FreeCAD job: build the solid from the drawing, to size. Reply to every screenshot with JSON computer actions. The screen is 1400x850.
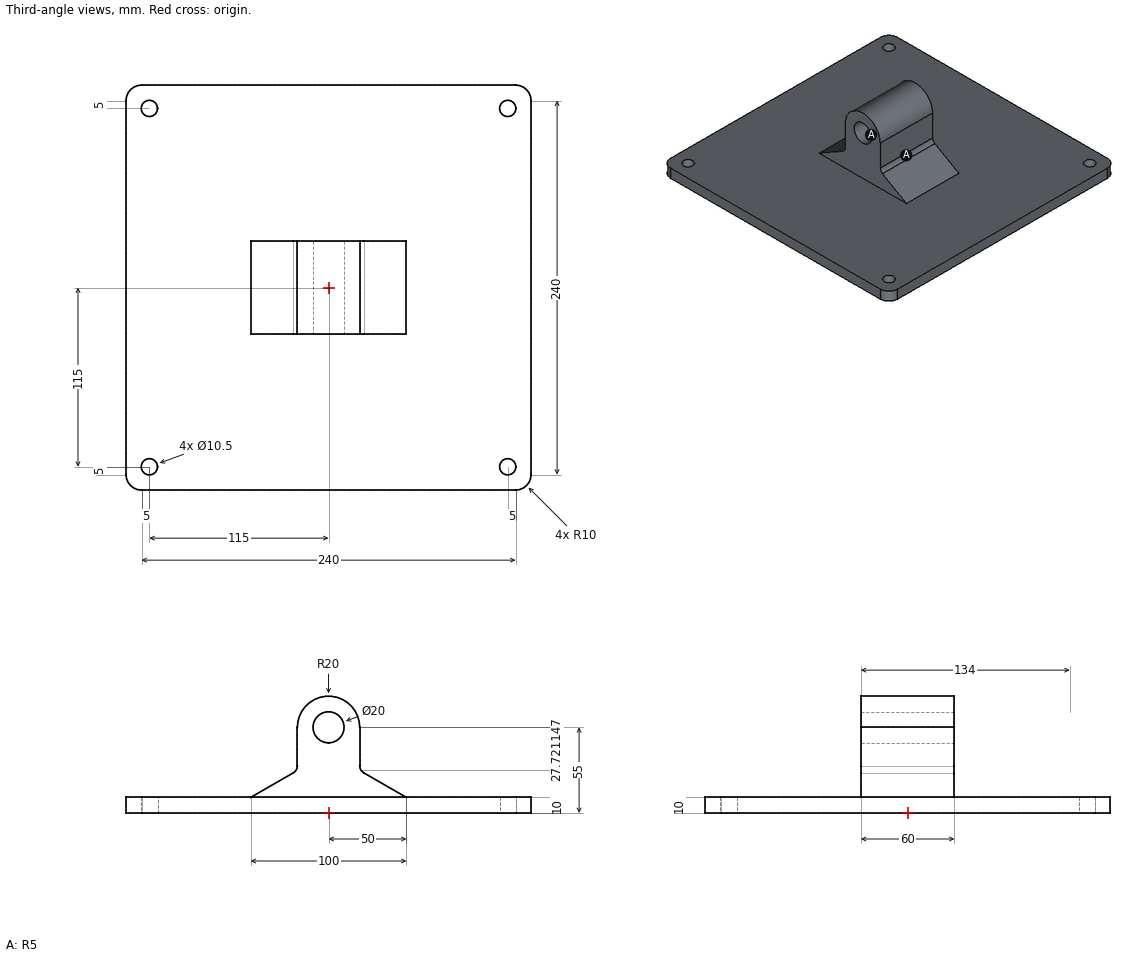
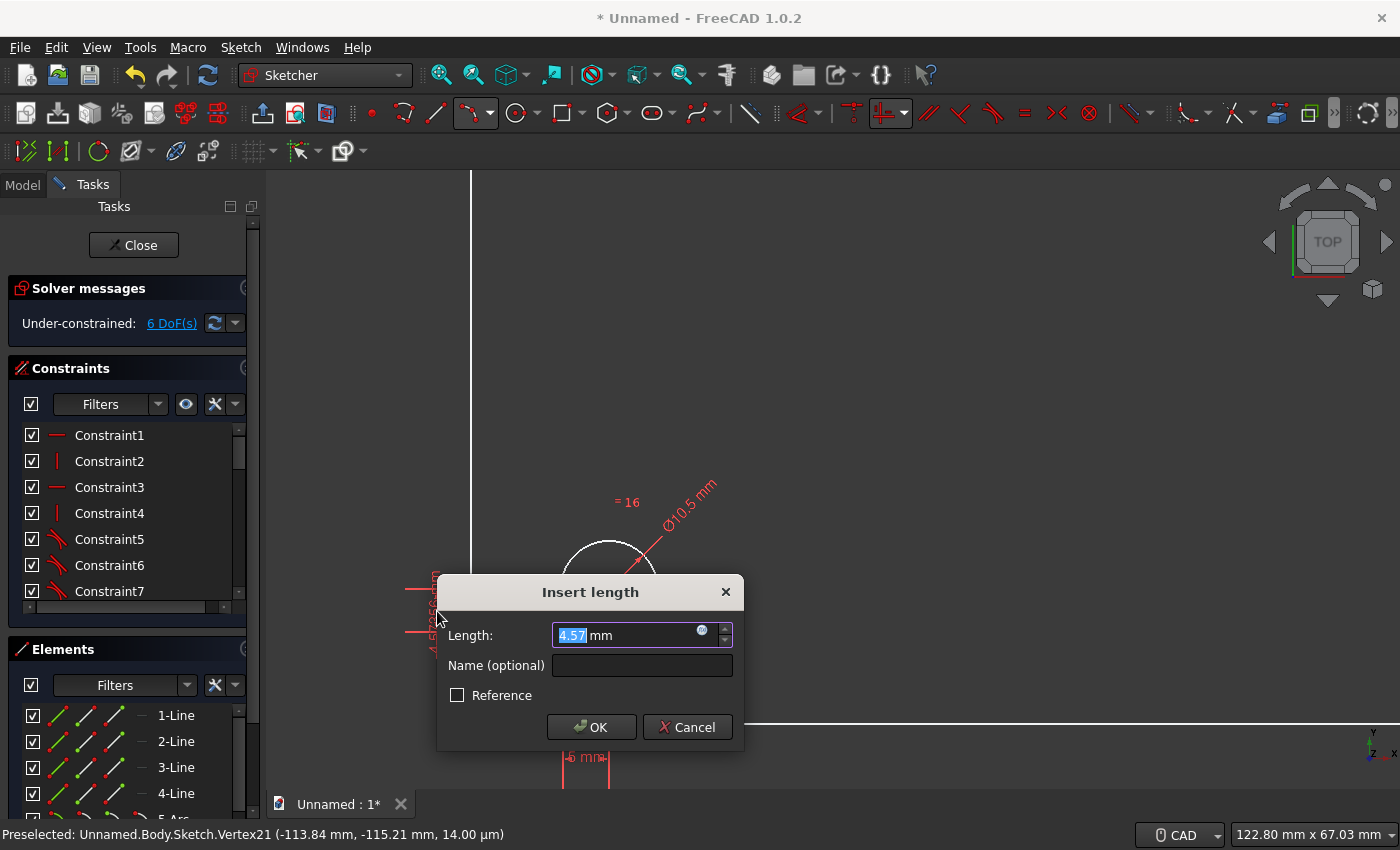
{"action": "type", "text": "5"}
{"action": "key", "text": "Return"}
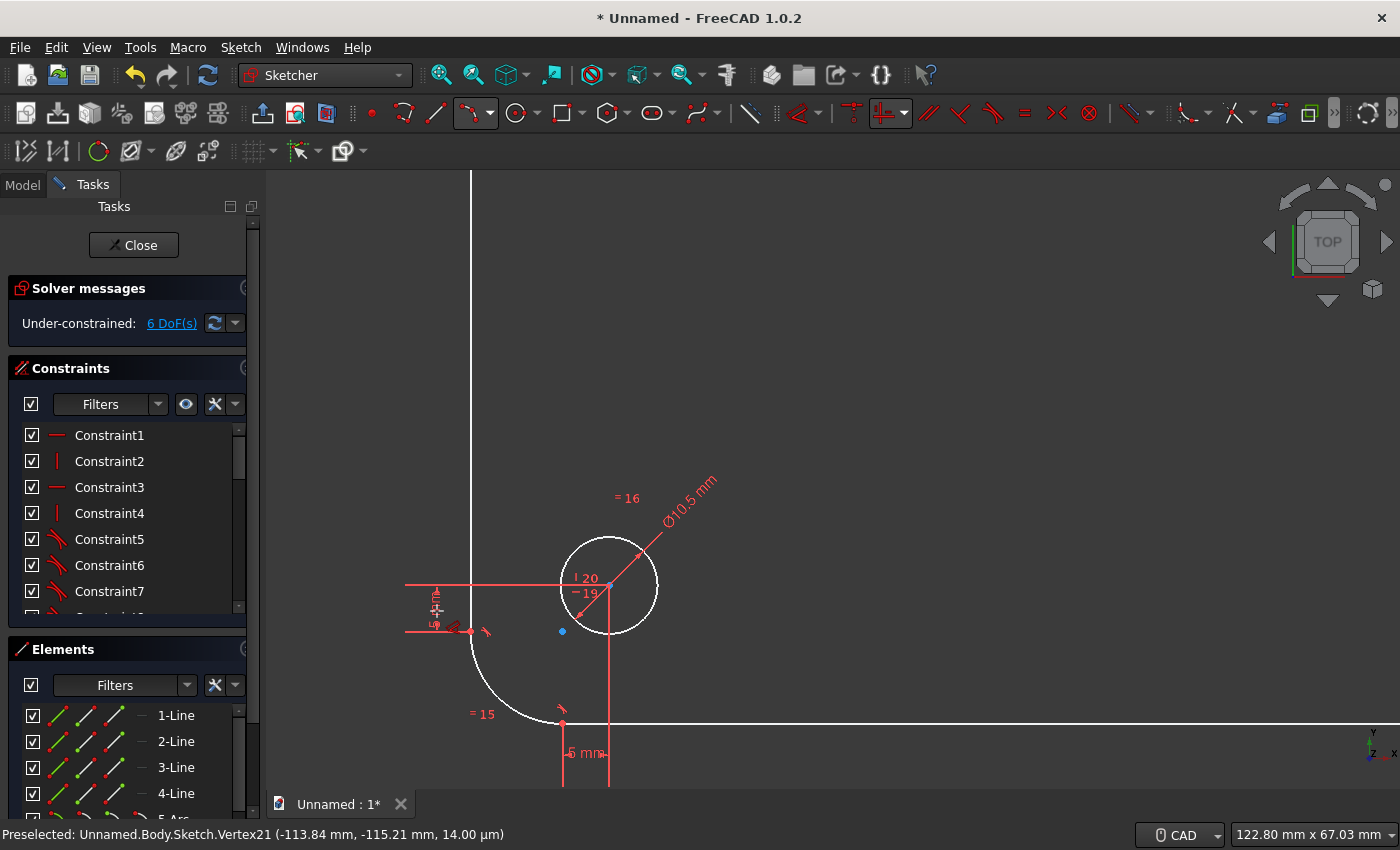
{"action": "scroll", "coordinate": [587, 668], "scroll_direction": "down", "scroll_amount": 9}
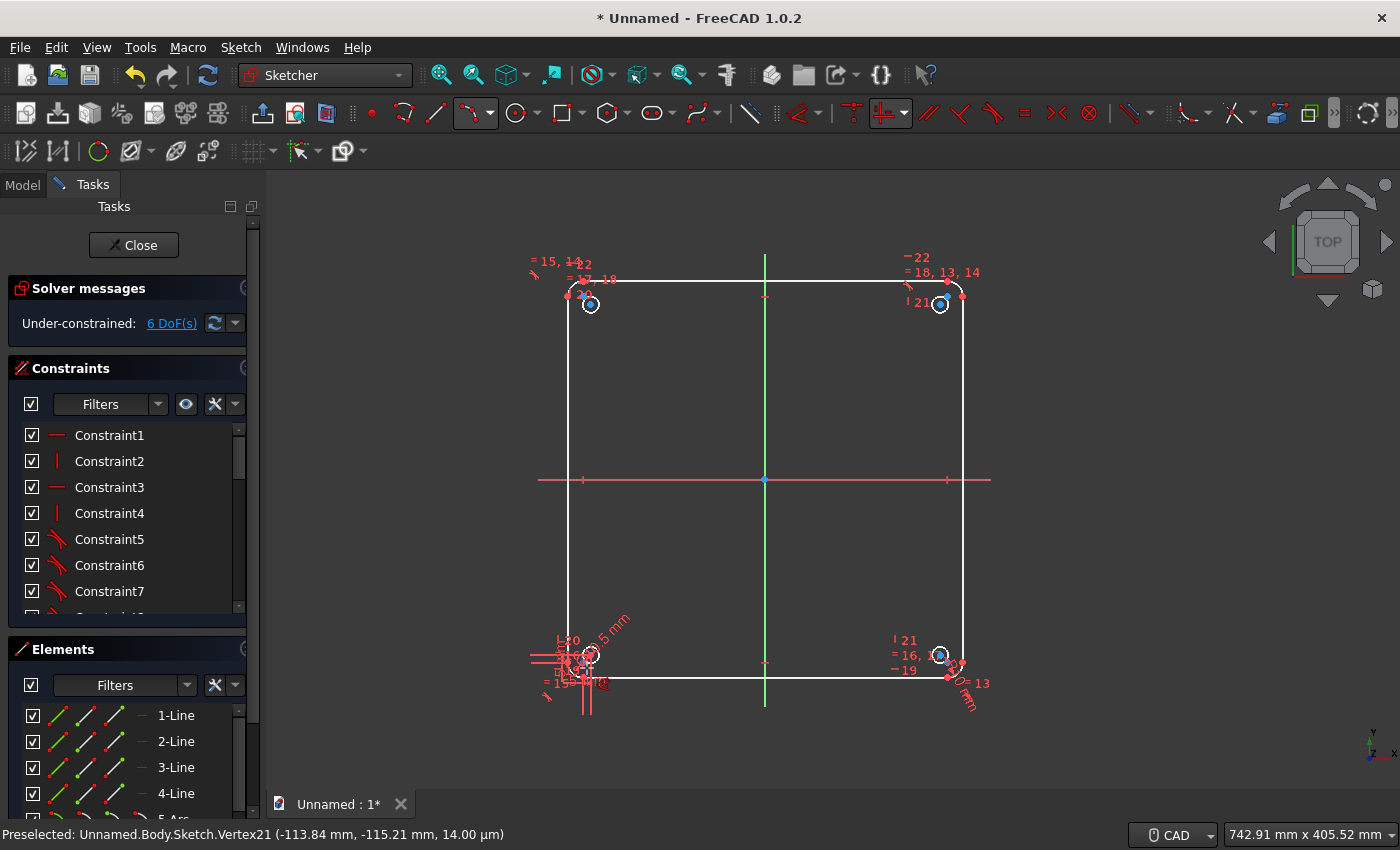
{"action": "scroll", "coordinate": [948, 678], "scroll_direction": "up", "scroll_amount": 9}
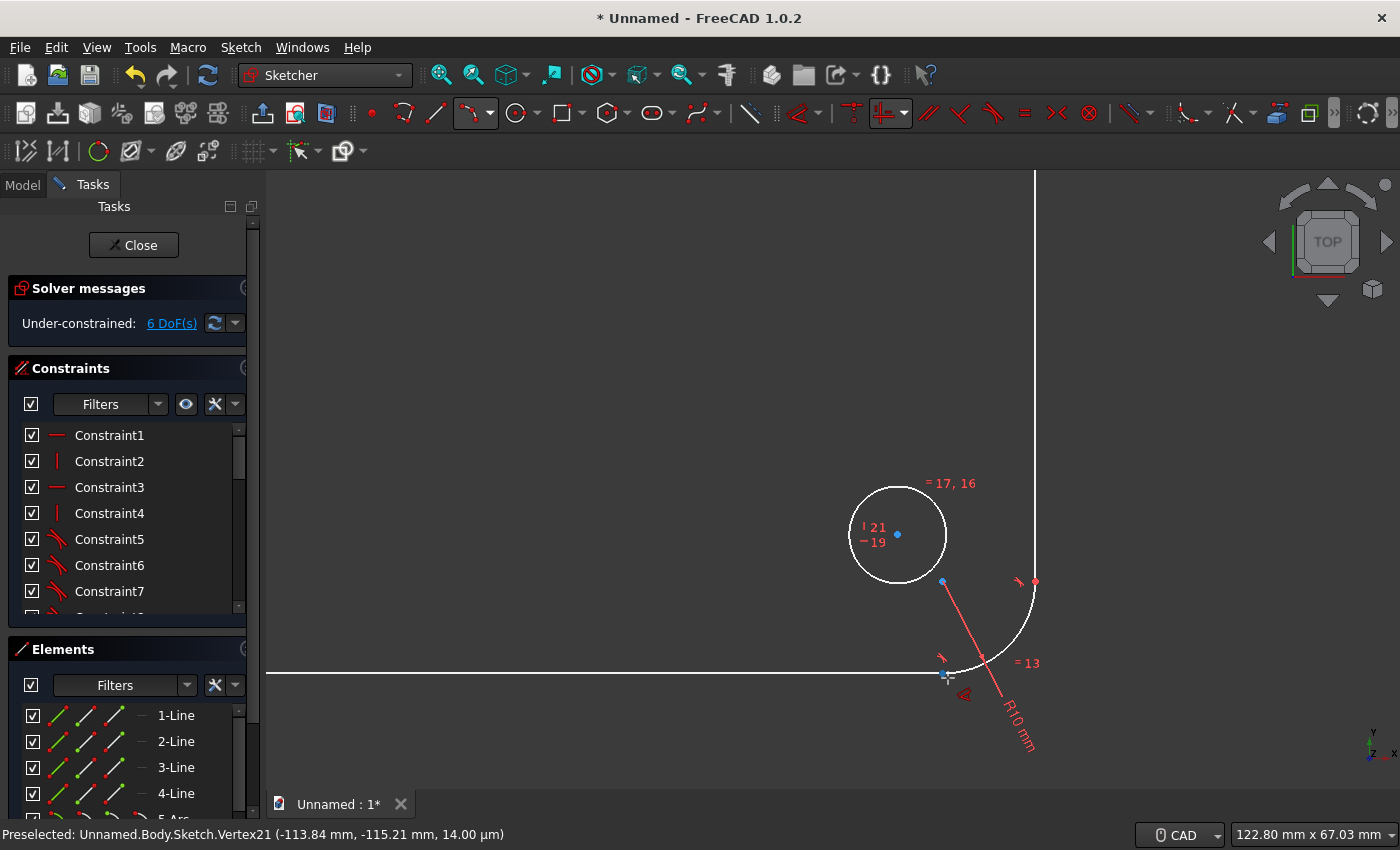
{"action": "left_click", "coordinate": [943, 673]}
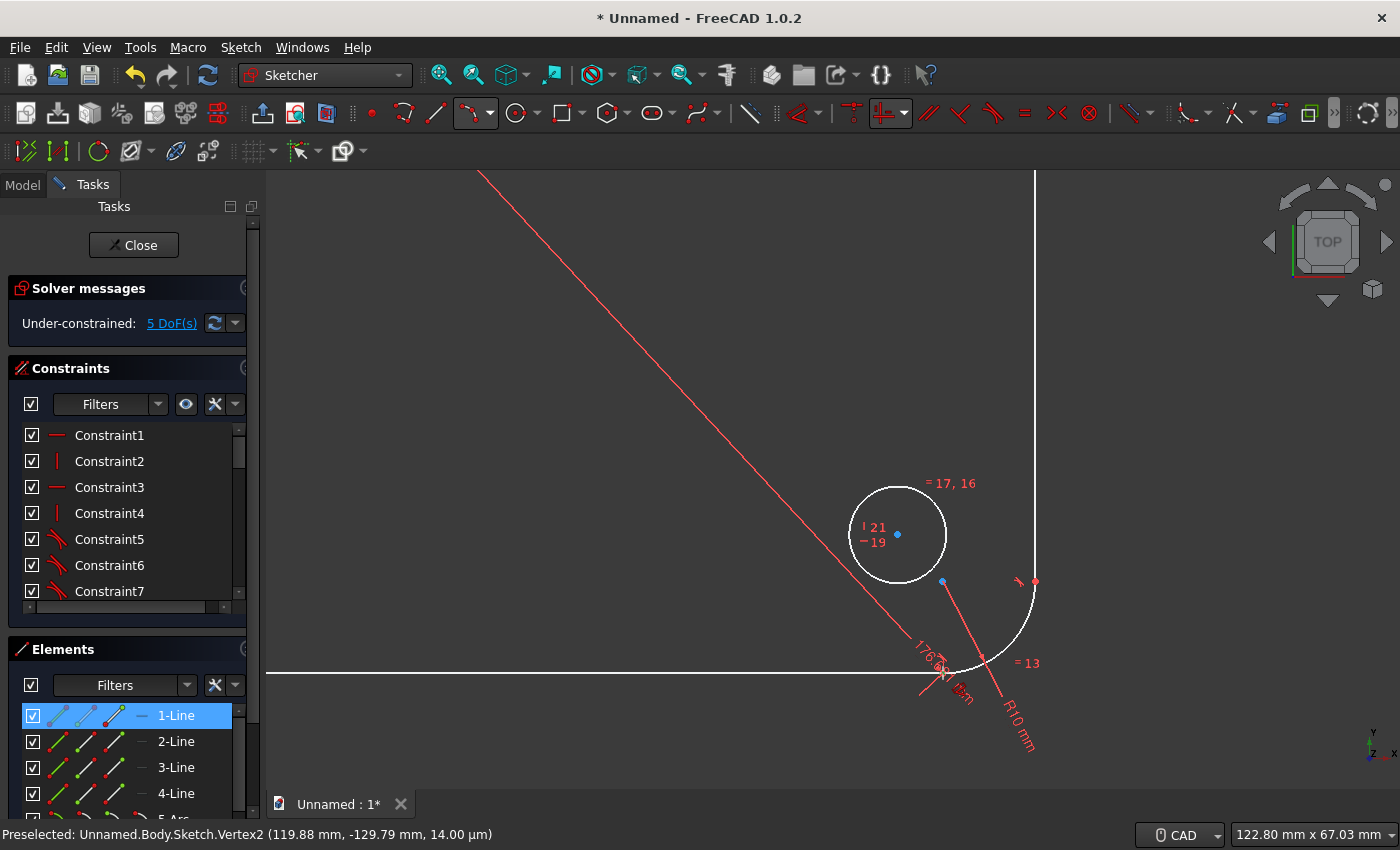
{"action": "left_click", "coordinate": [898, 535]}
{"action": "left_click", "coordinate": [920, 707]}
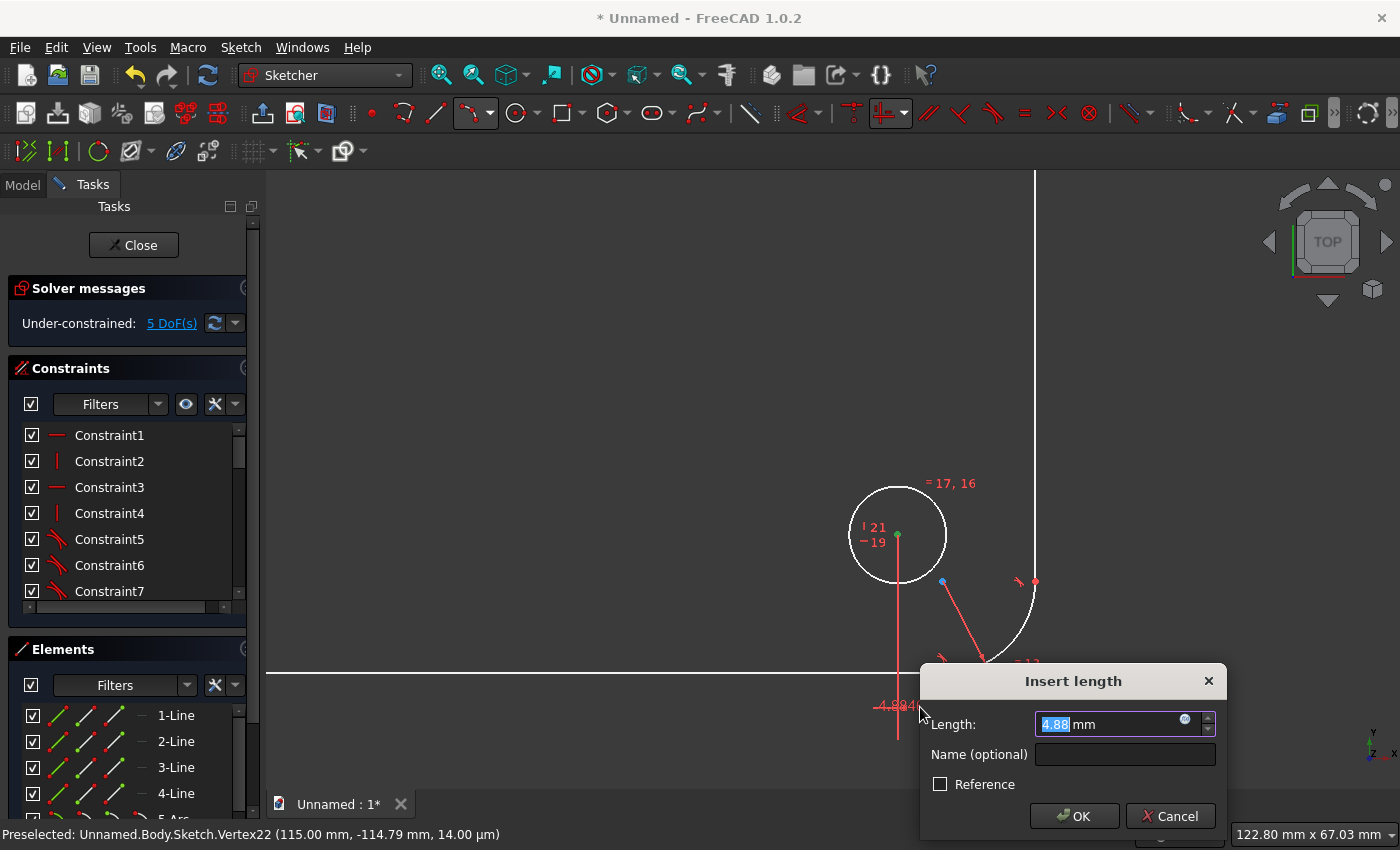
{"action": "type", "text": "5"}
{"action": "key", "text": "Return"}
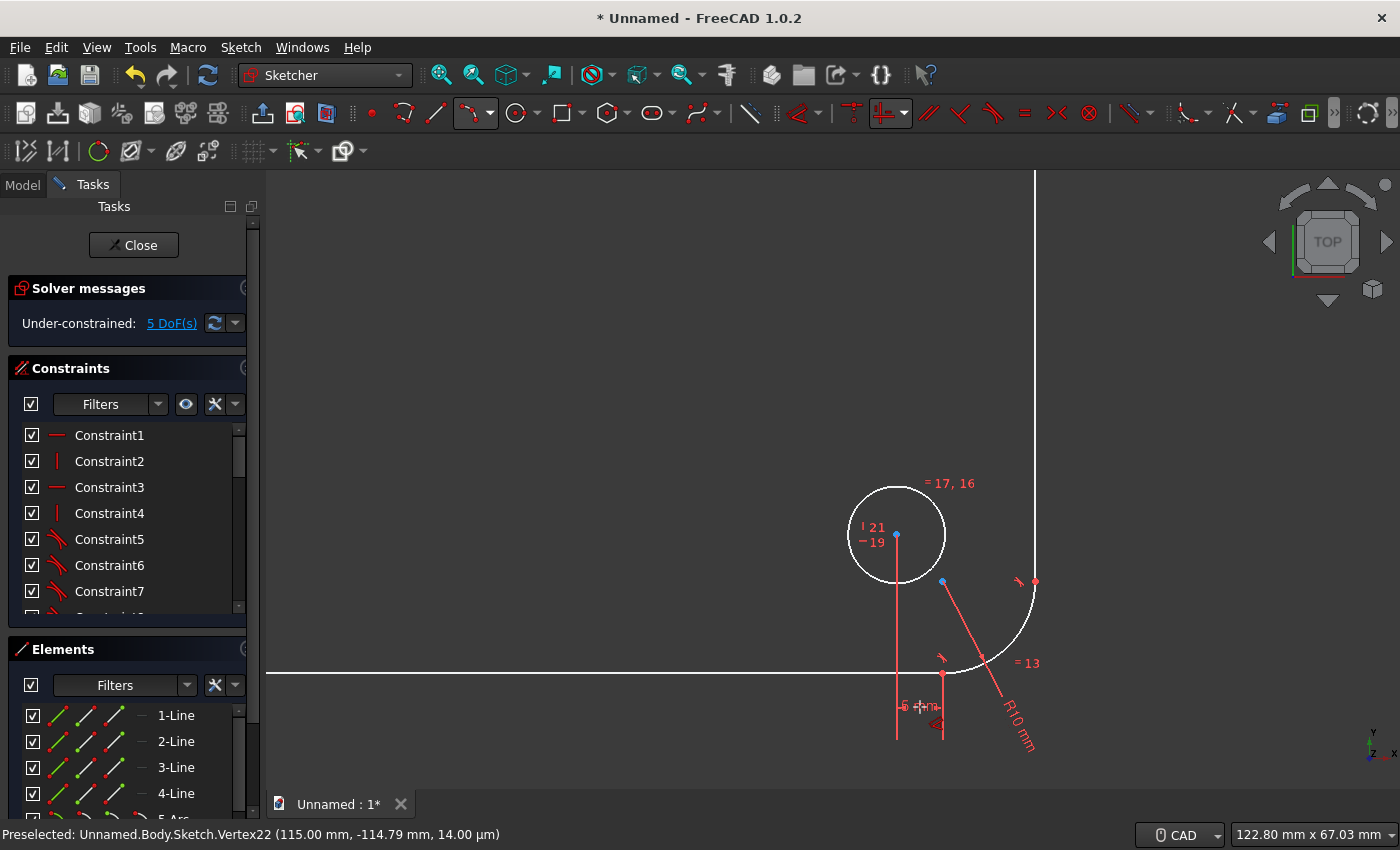
{"action": "scroll", "coordinate": [948, 678], "scroll_direction": "down", "scroll_amount": 9}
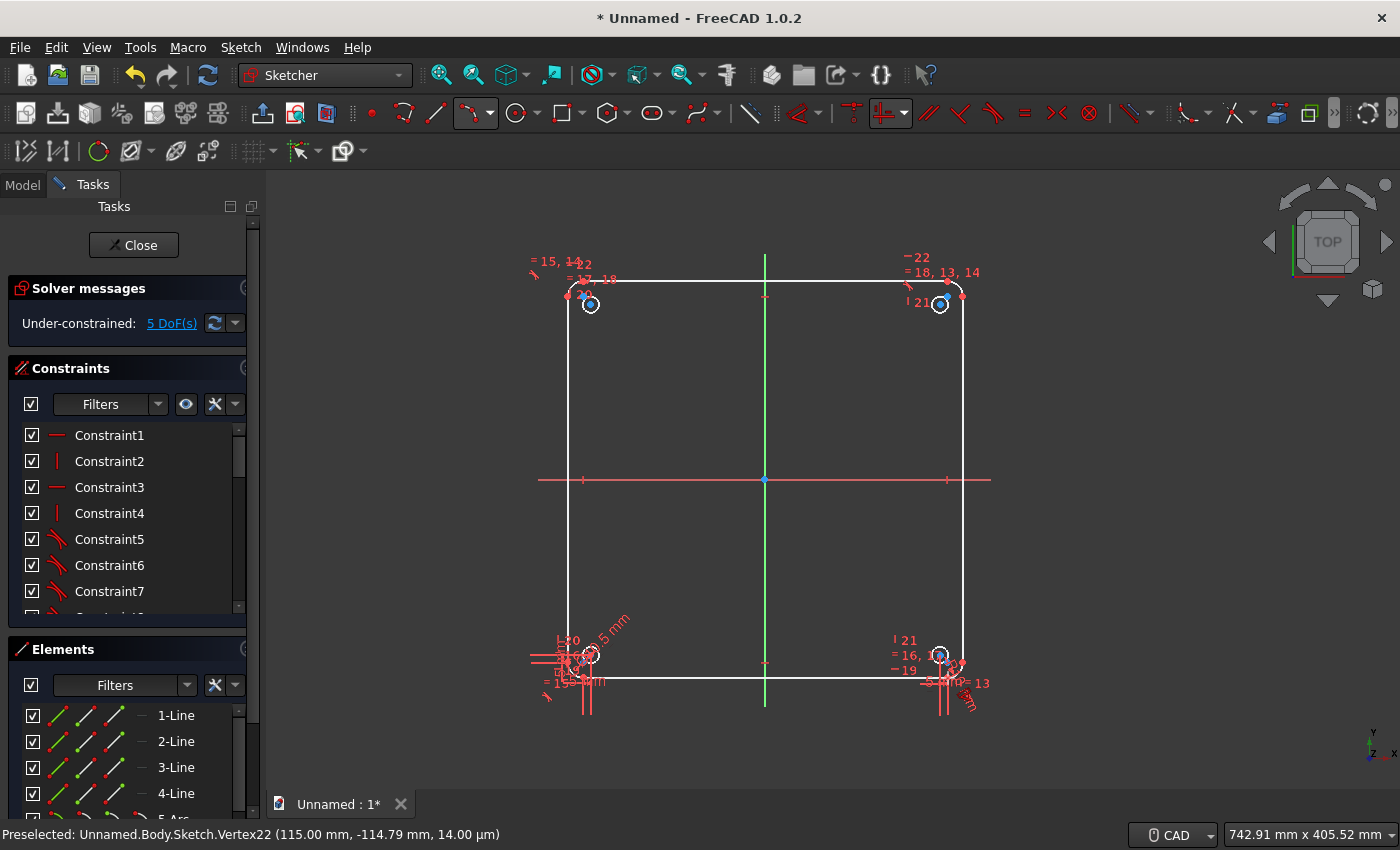
{"action": "scroll", "coordinate": [568, 297], "scroll_direction": "up", "scroll_amount": 9}